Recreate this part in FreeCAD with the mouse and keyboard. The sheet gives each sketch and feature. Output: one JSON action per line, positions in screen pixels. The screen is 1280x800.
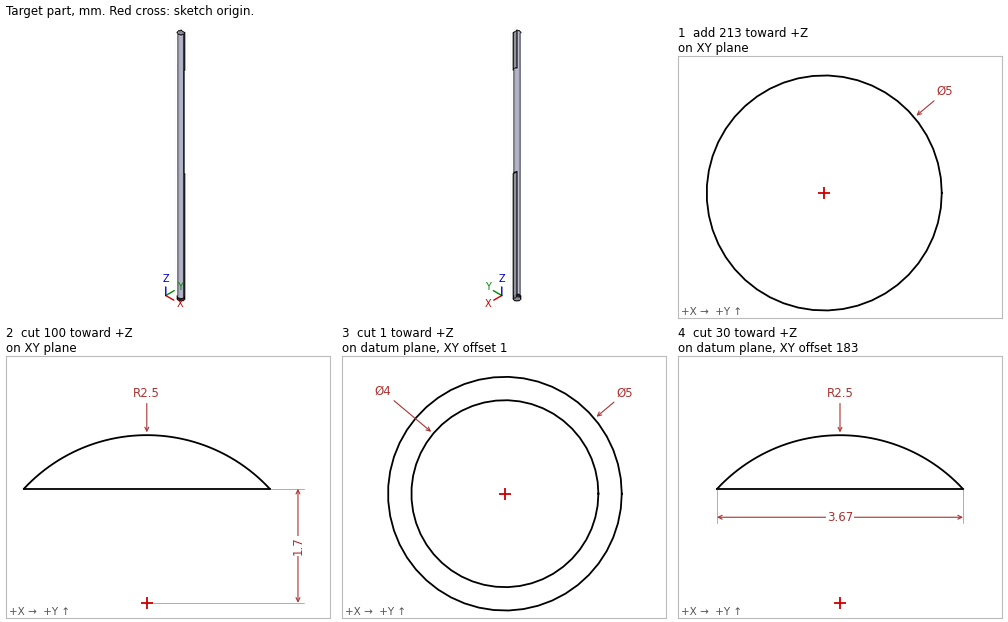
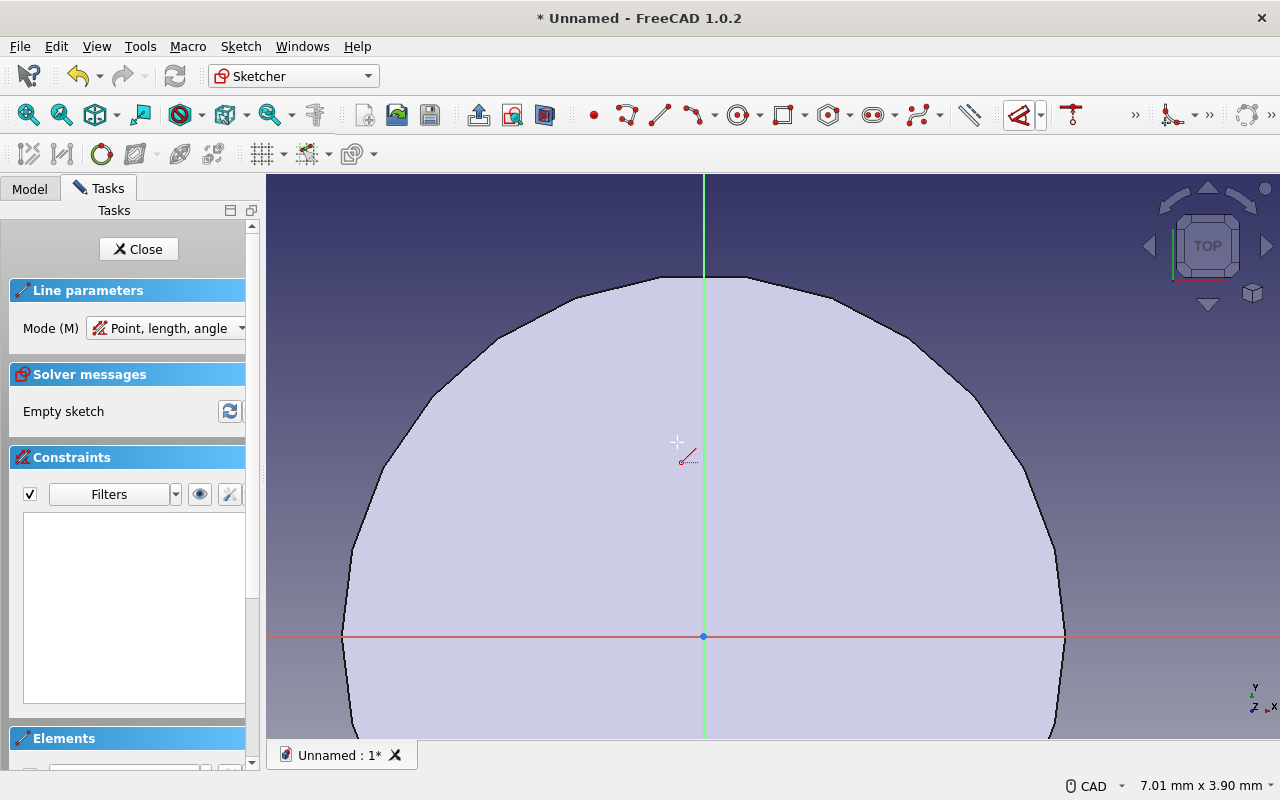
{"action": "left_click", "coordinate": [969, 390]}
{"action": "left_click", "coordinate": [438, 390]}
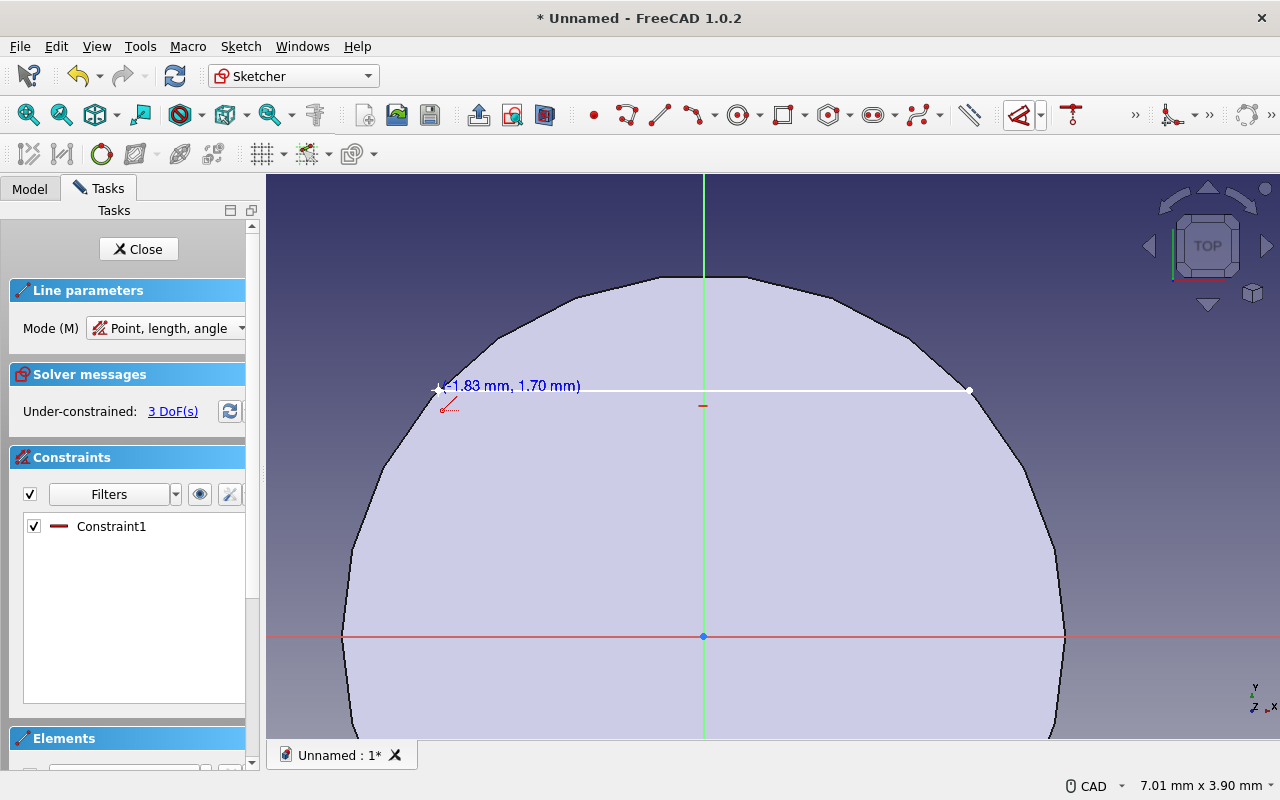
{"action": "key", "text": "g 3 a"}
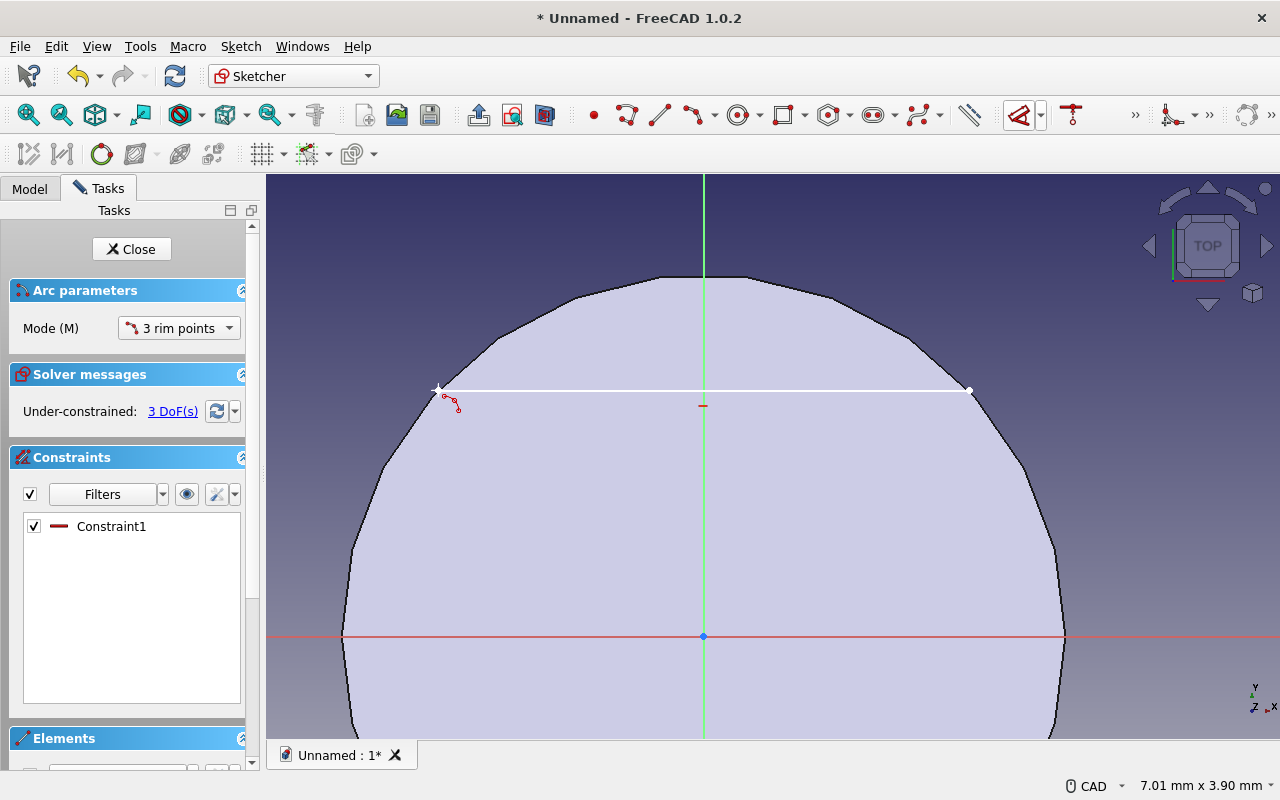
{"action": "left_click", "coordinate": [438, 391]}
{"action": "left_click", "coordinate": [969, 391]}
{"action": "left_click", "coordinate": [763, 280]}
{"action": "key", "text": "Escape"}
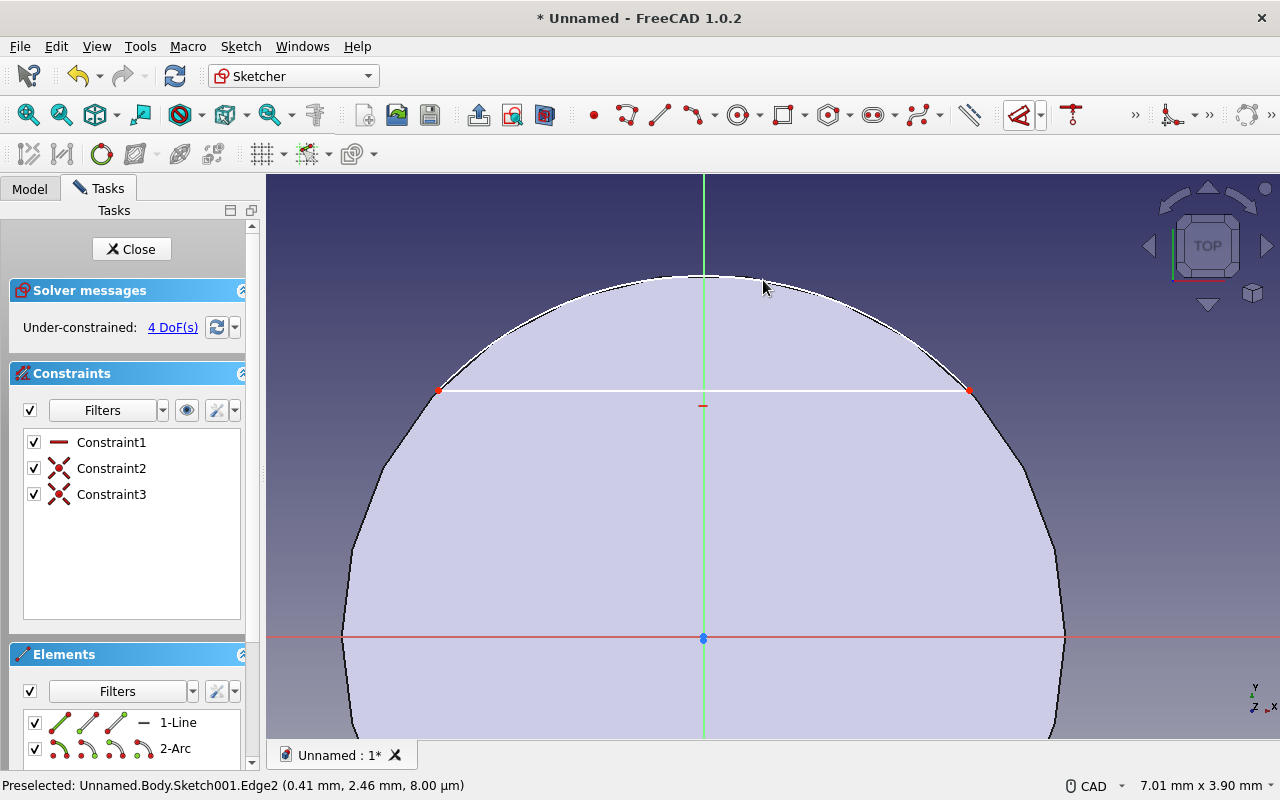
{"action": "left_click_drag", "start_coordinate": [694, 627], "coordinate": [714, 650]}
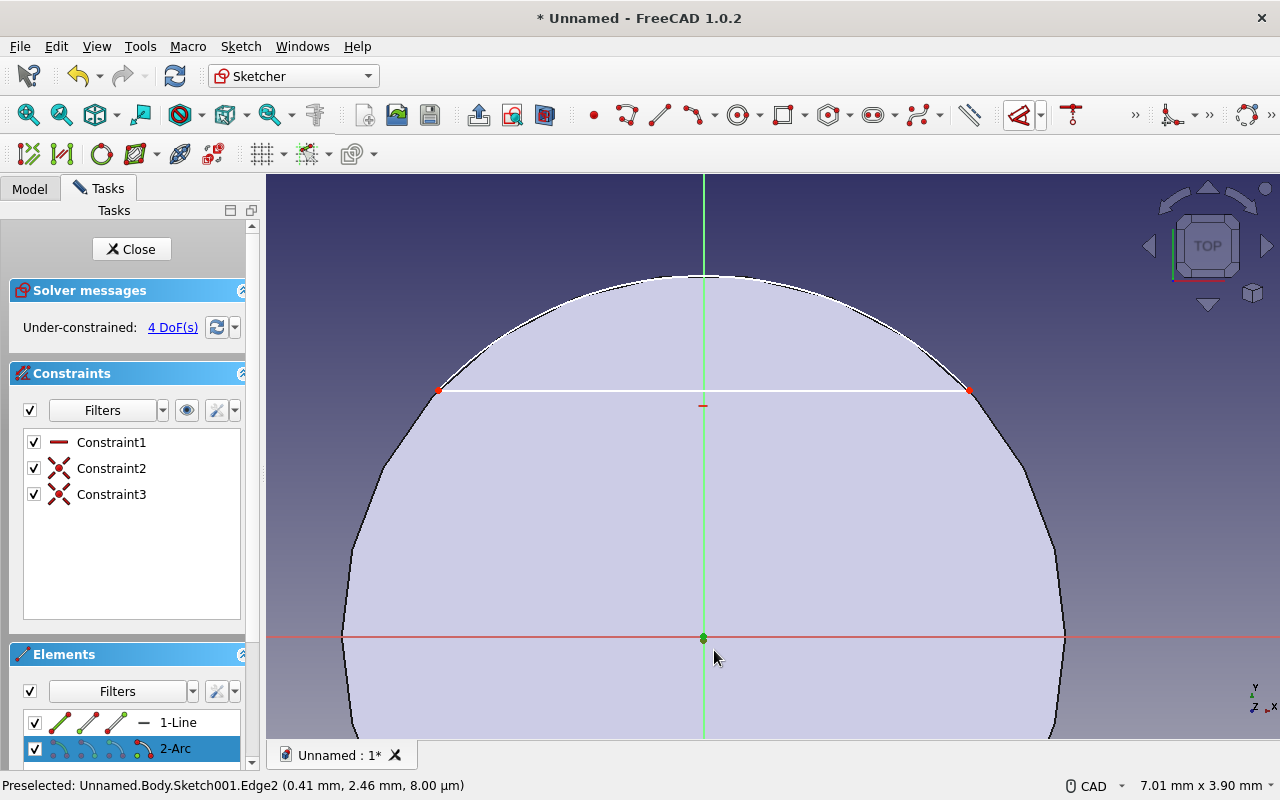
{"action": "key", "text": "c"}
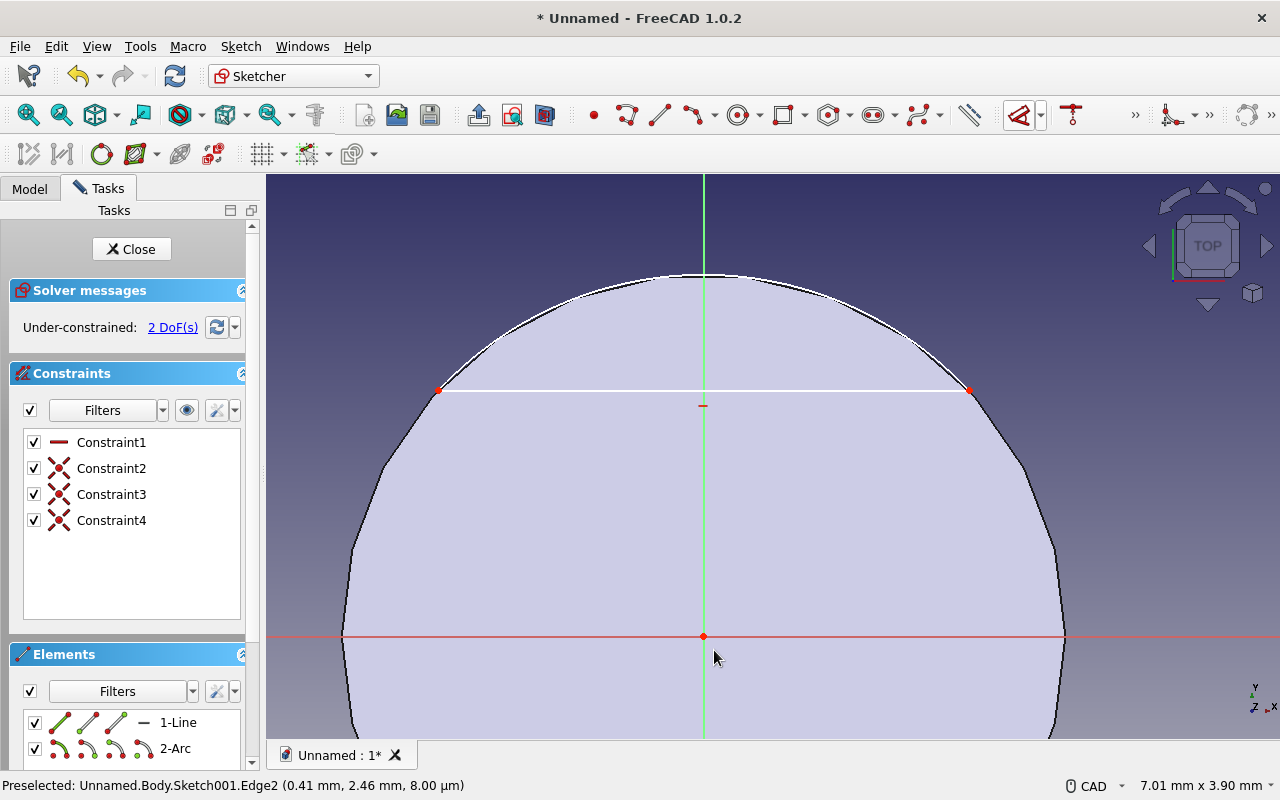
{"action": "left_click", "coordinate": [821, 294]}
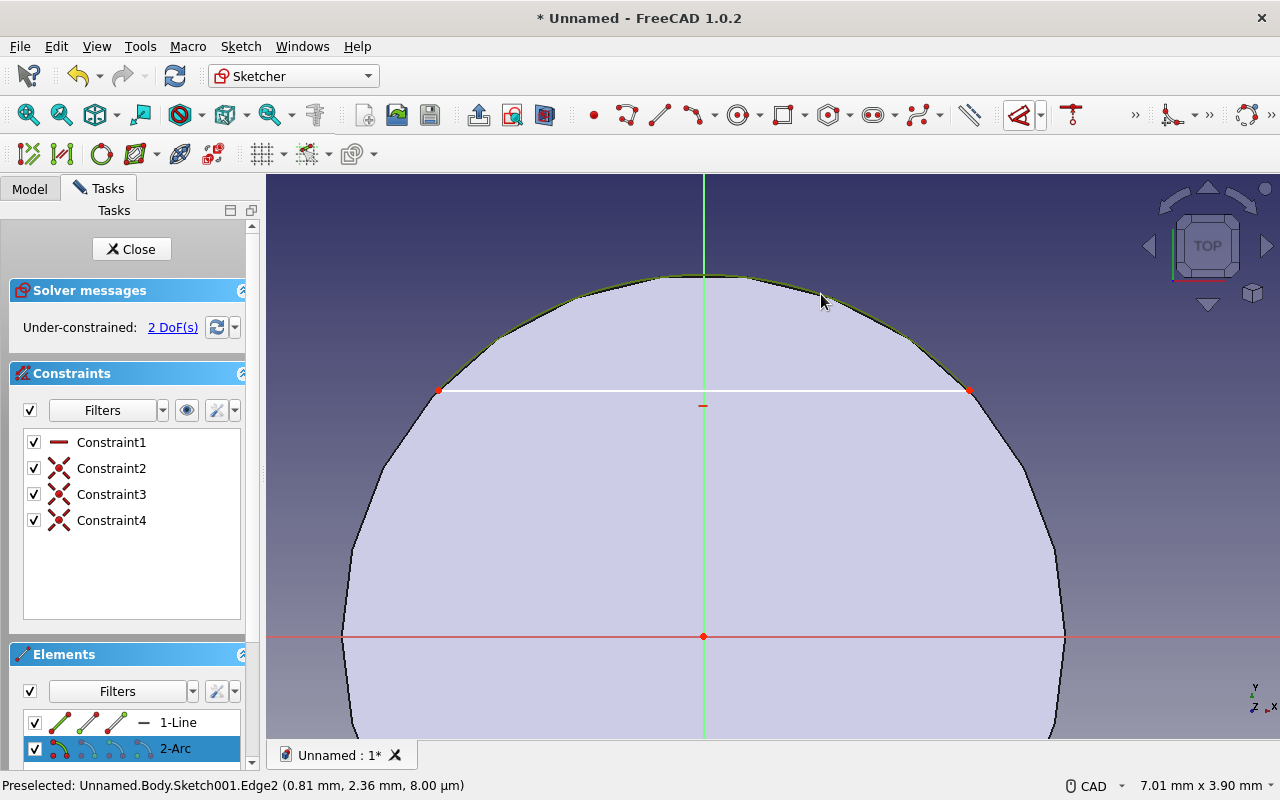
{"action": "key", "text": "k r"}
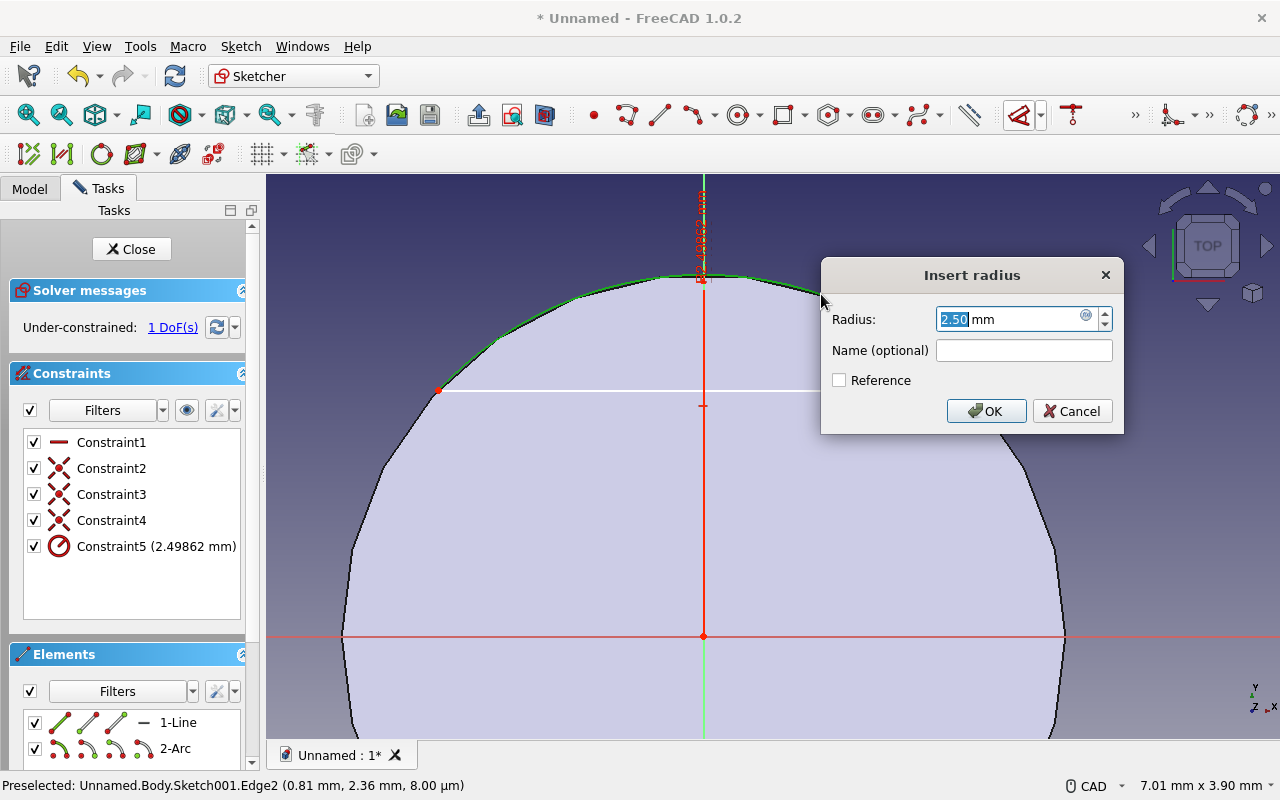
{"action": "type", "text": "2.5"}
{"action": "key", "text": "Return"}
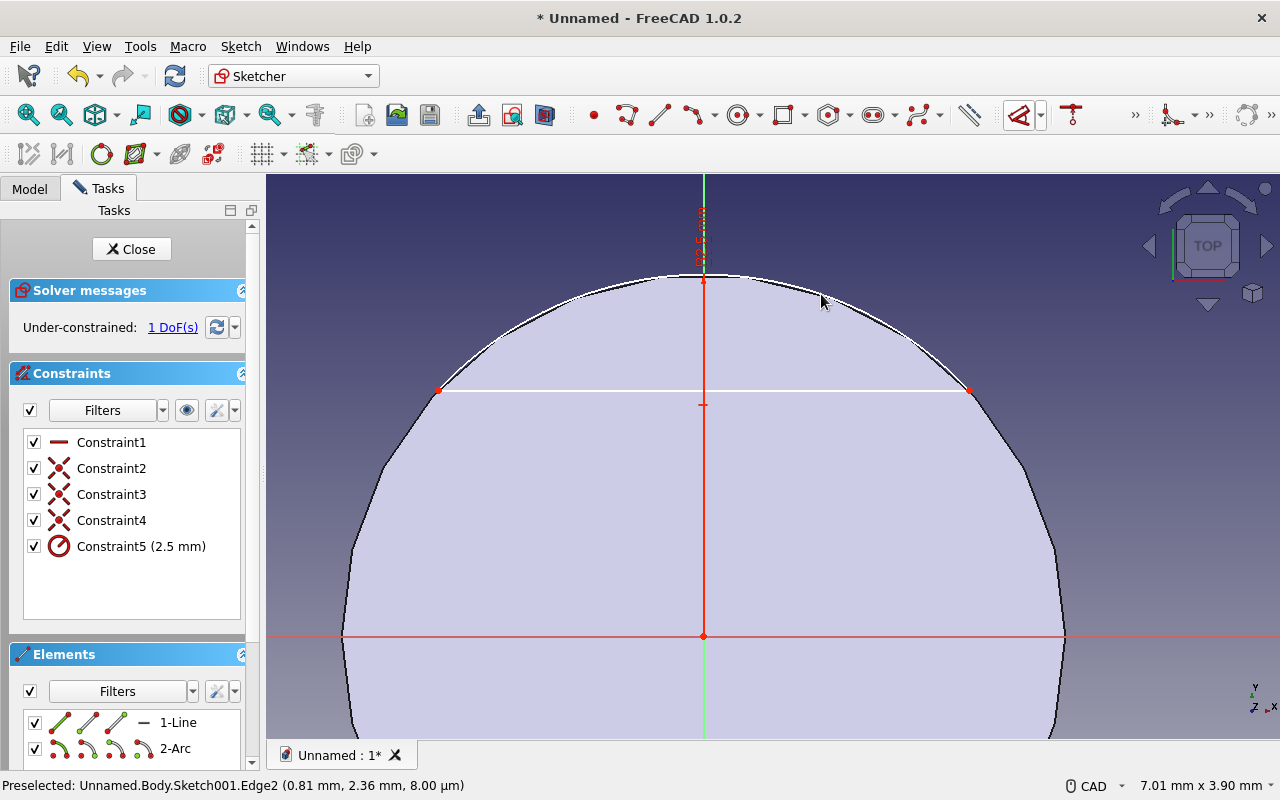
{"action": "left_click", "coordinate": [969, 391]}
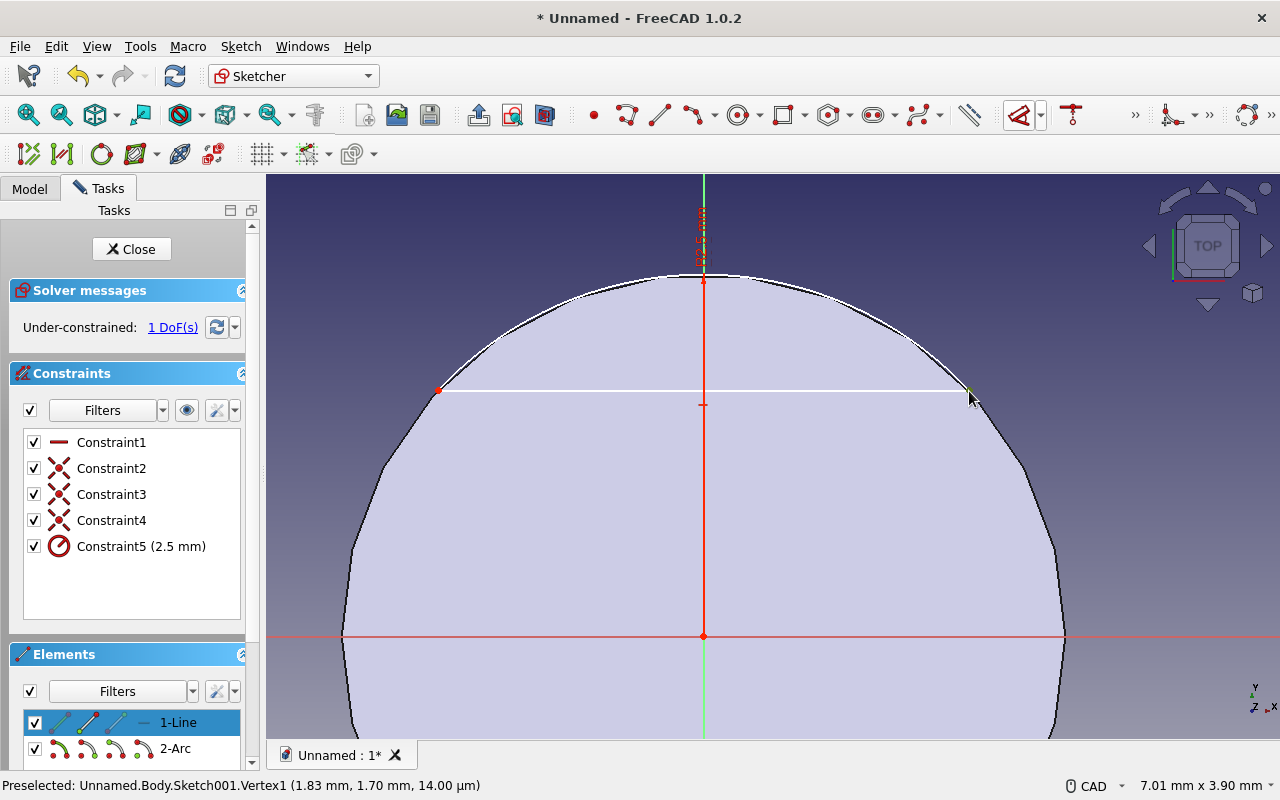
{"action": "key", "text": "i"}